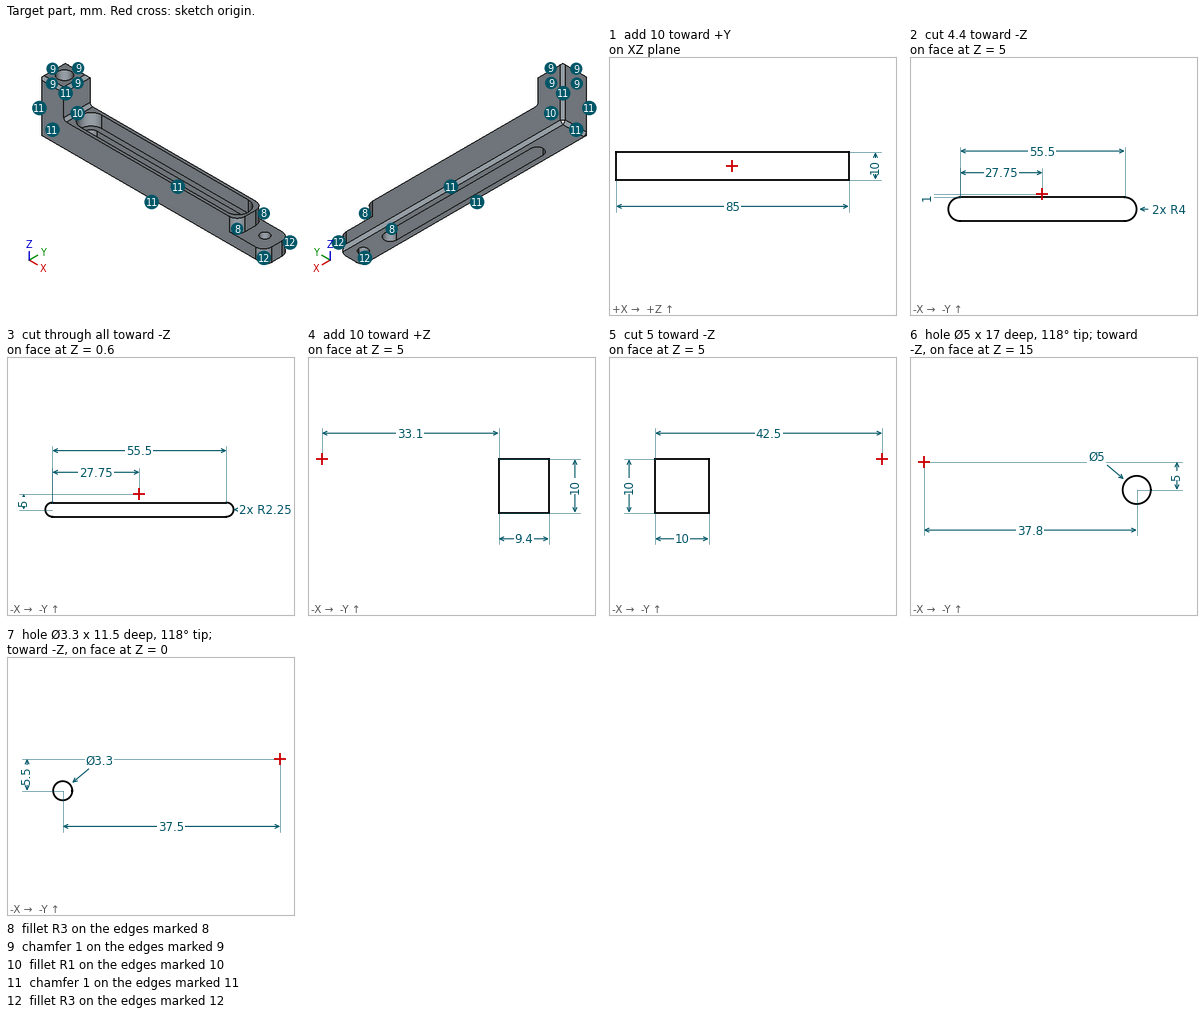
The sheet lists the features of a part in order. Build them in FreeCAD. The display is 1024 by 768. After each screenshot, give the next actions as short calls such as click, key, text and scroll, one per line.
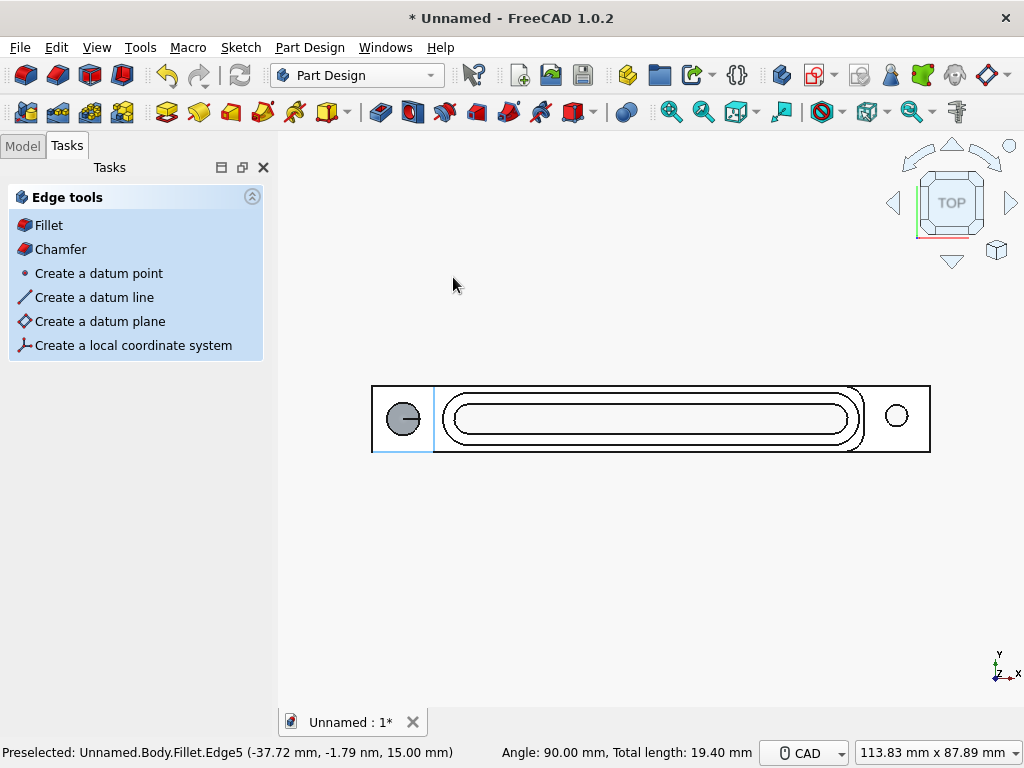
click(403, 385, ctrl)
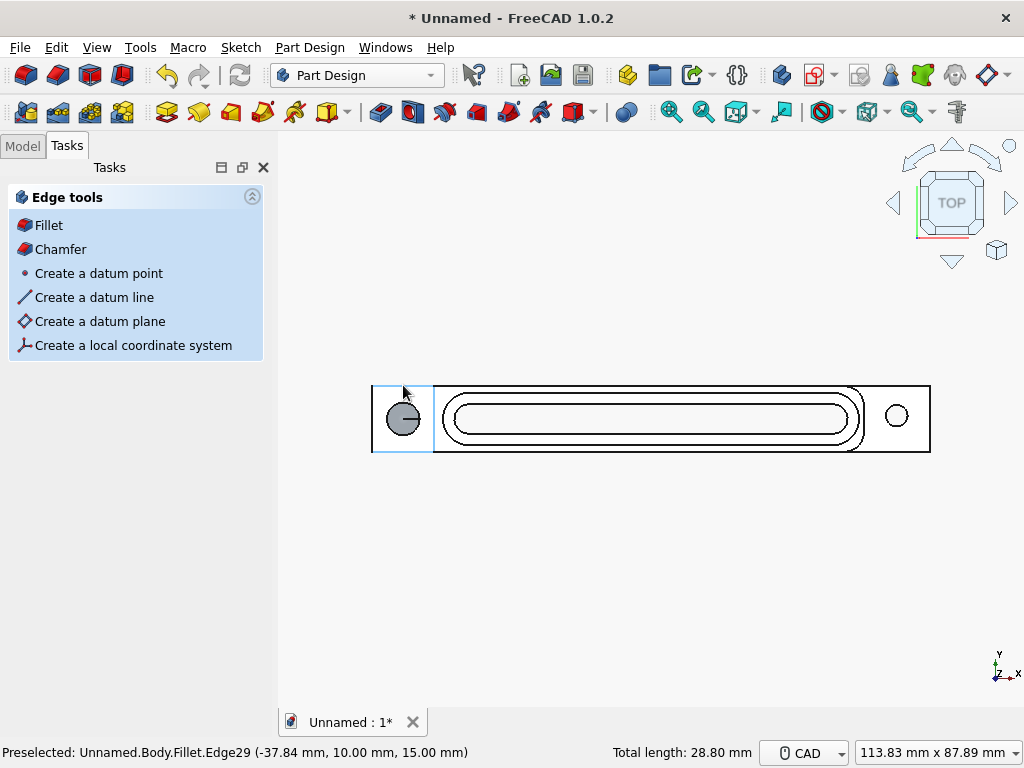
click(372, 418, ctrl)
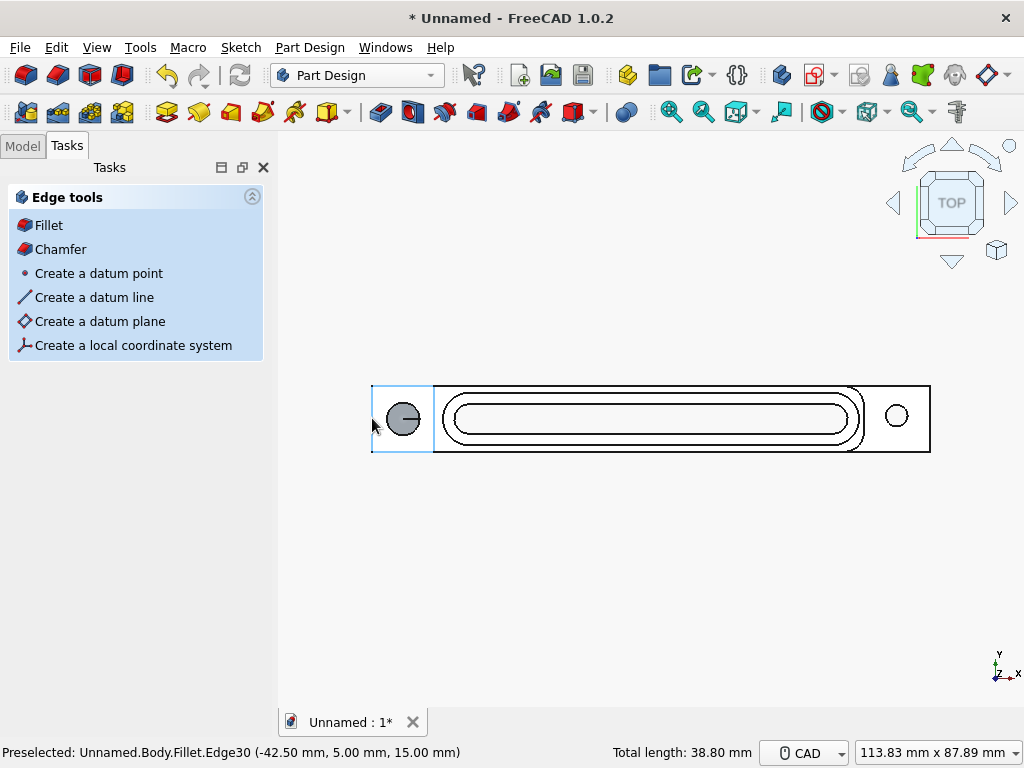
click(58, 76)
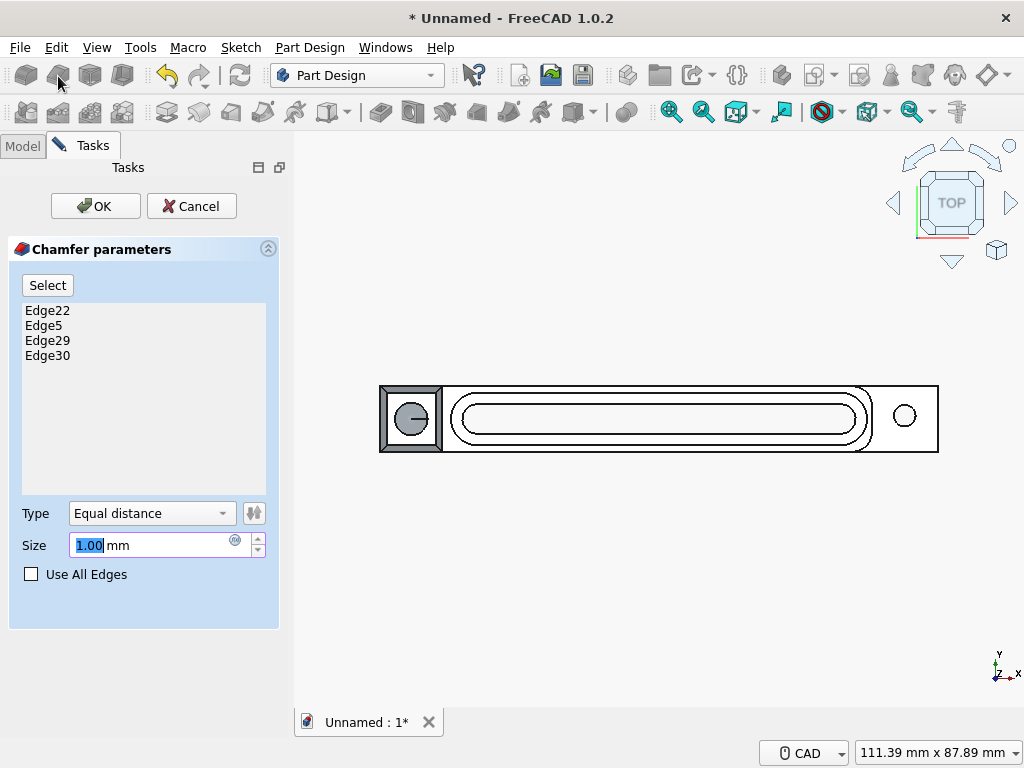
text(1)
key(Tab)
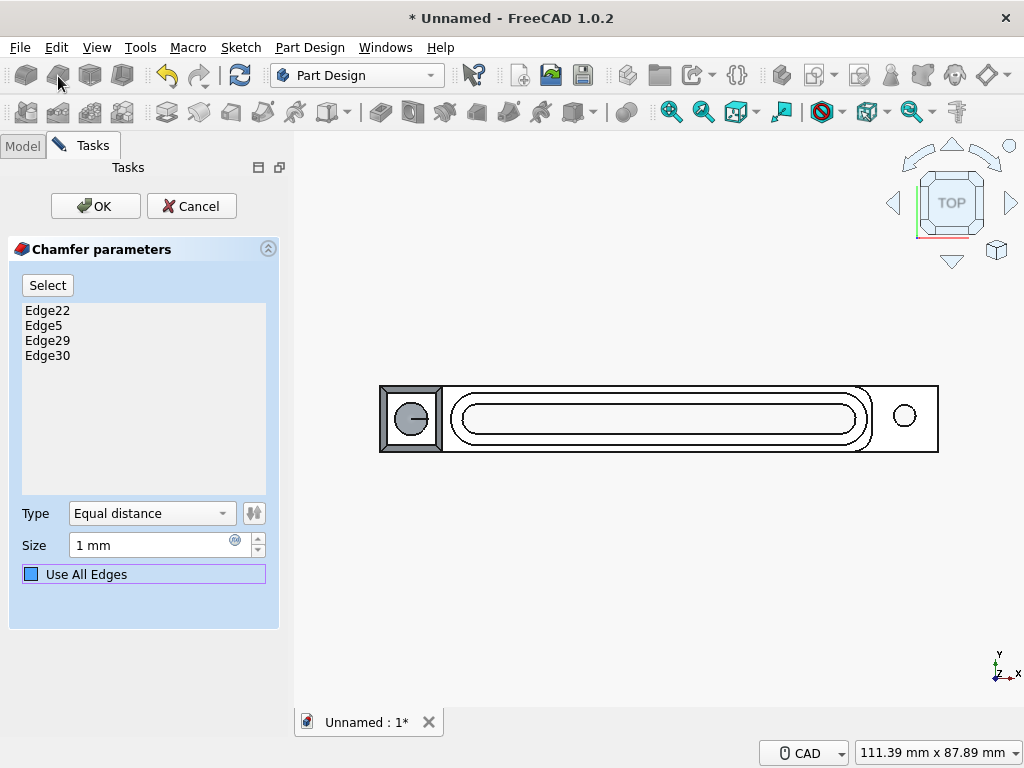
click(96, 206)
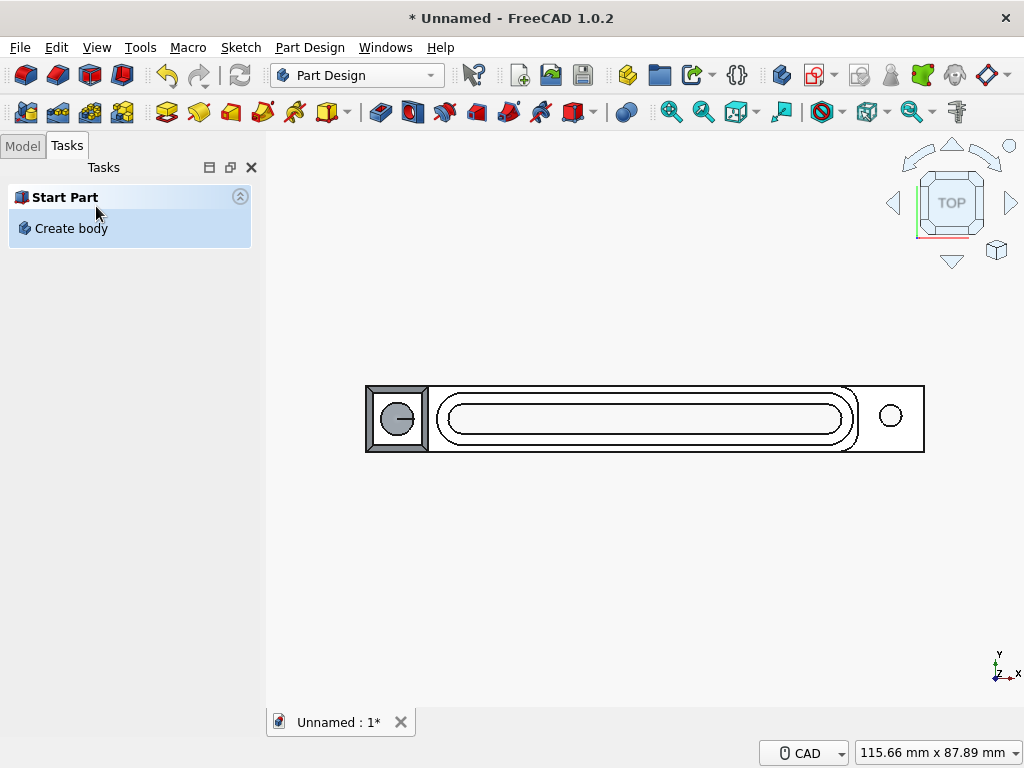
key(0)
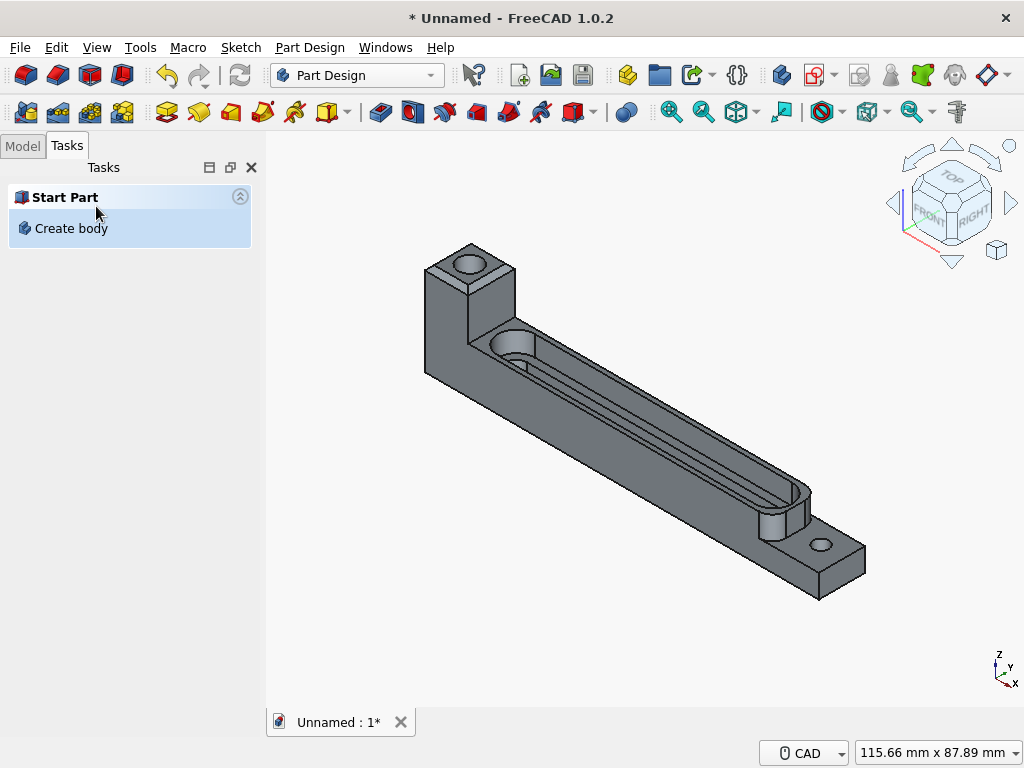
key(2)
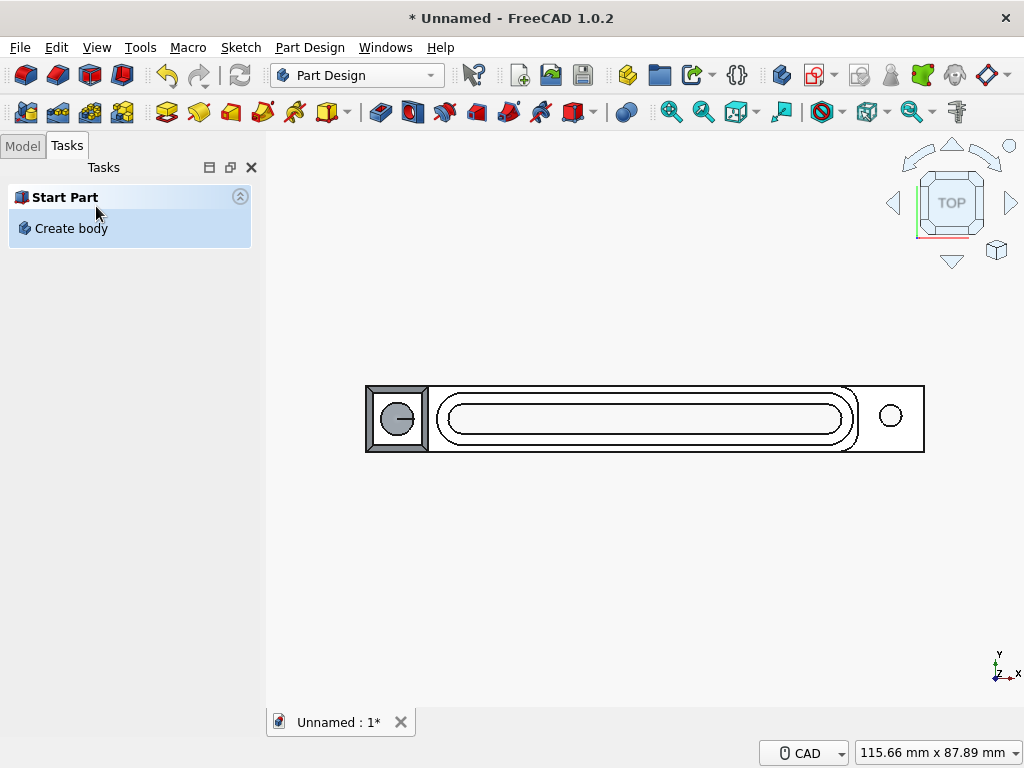
key(1)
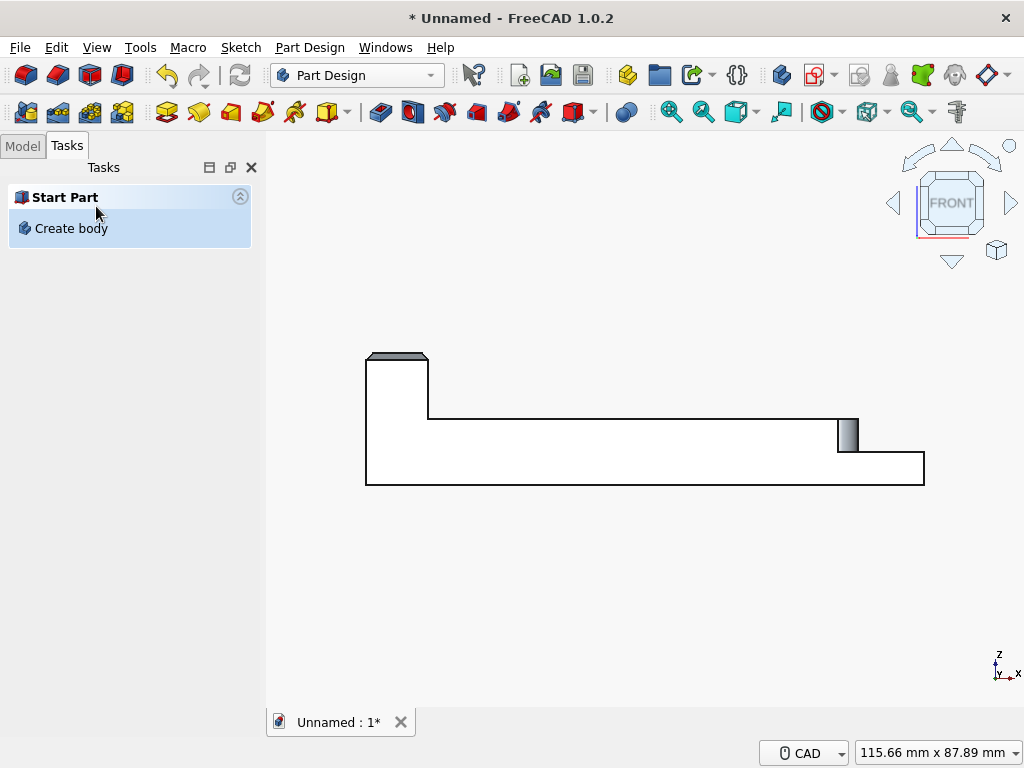
key(3)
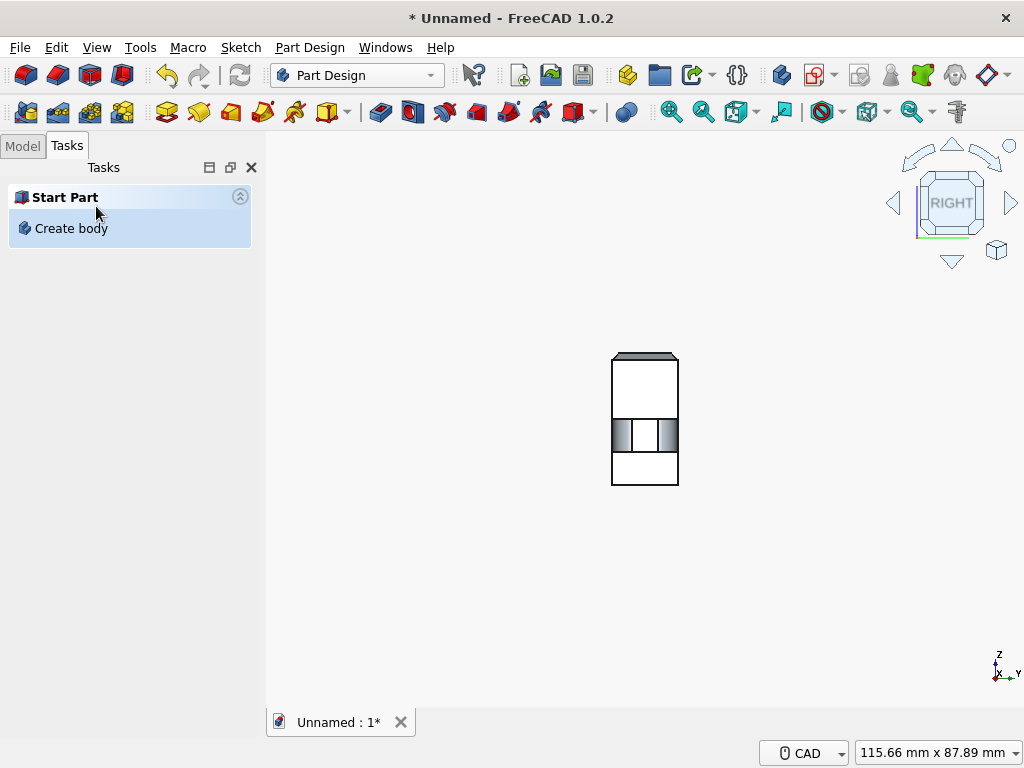
key(v)
key(f)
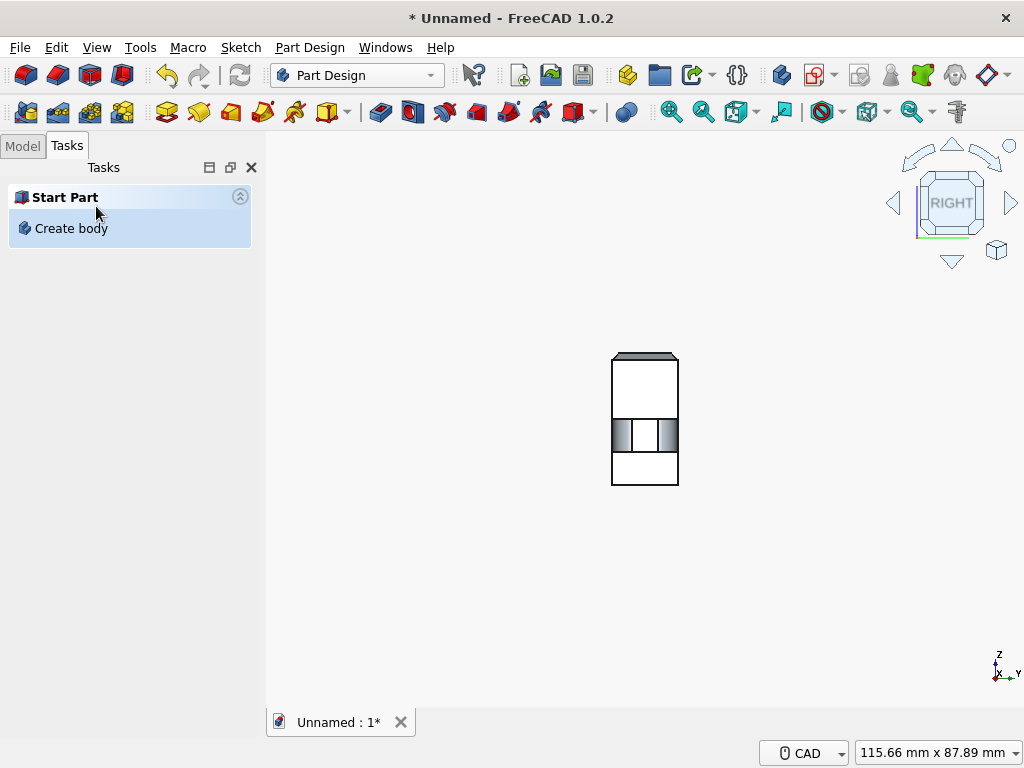
key(5)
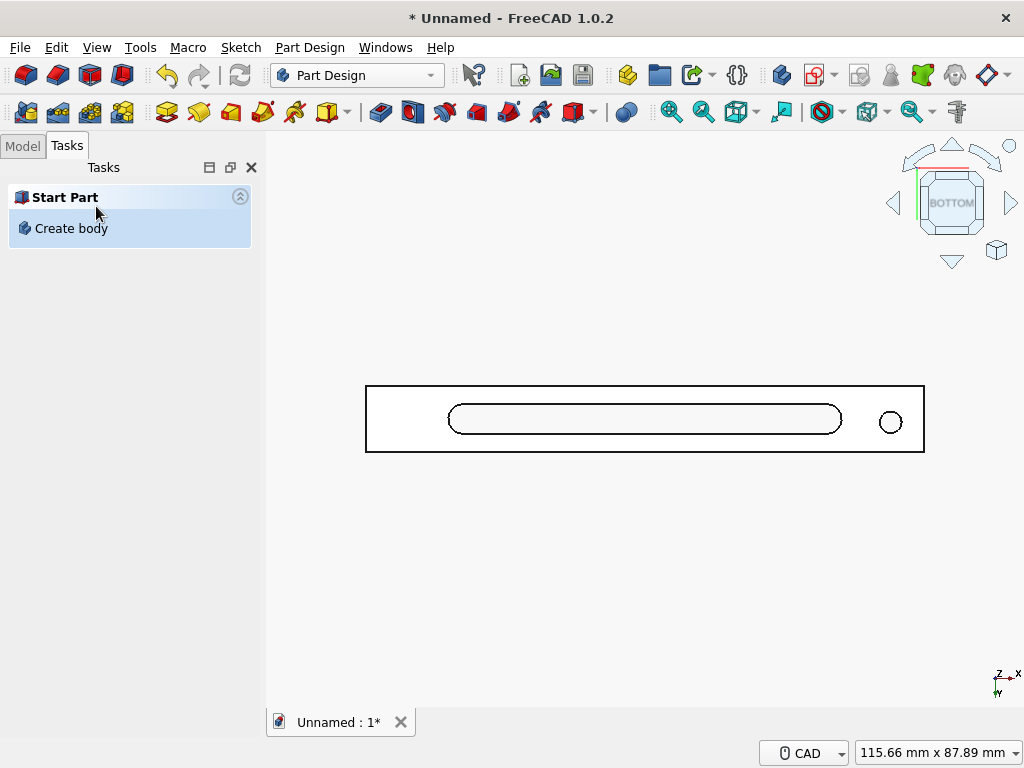
key(4)